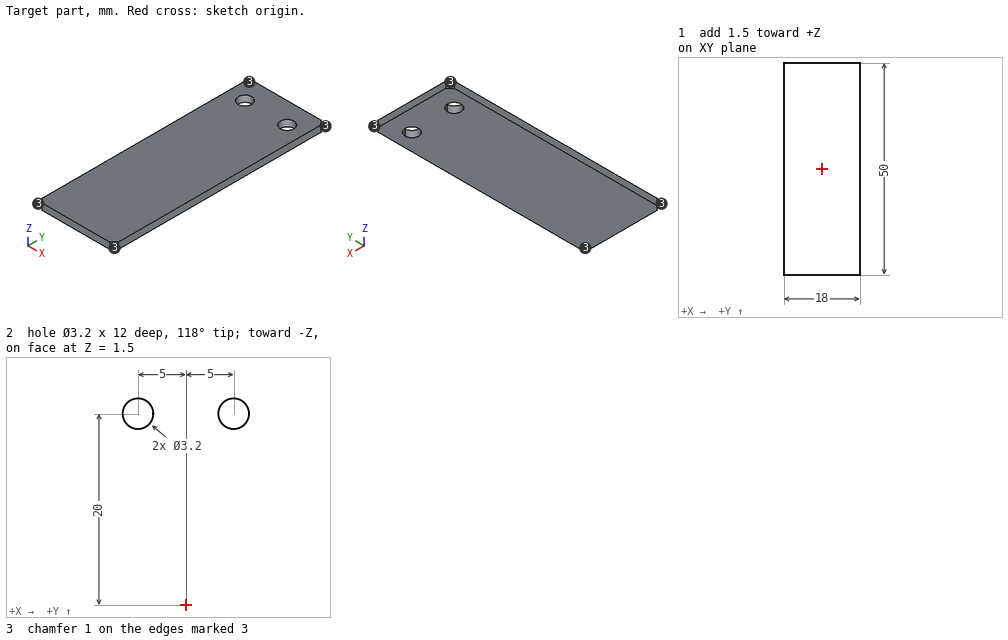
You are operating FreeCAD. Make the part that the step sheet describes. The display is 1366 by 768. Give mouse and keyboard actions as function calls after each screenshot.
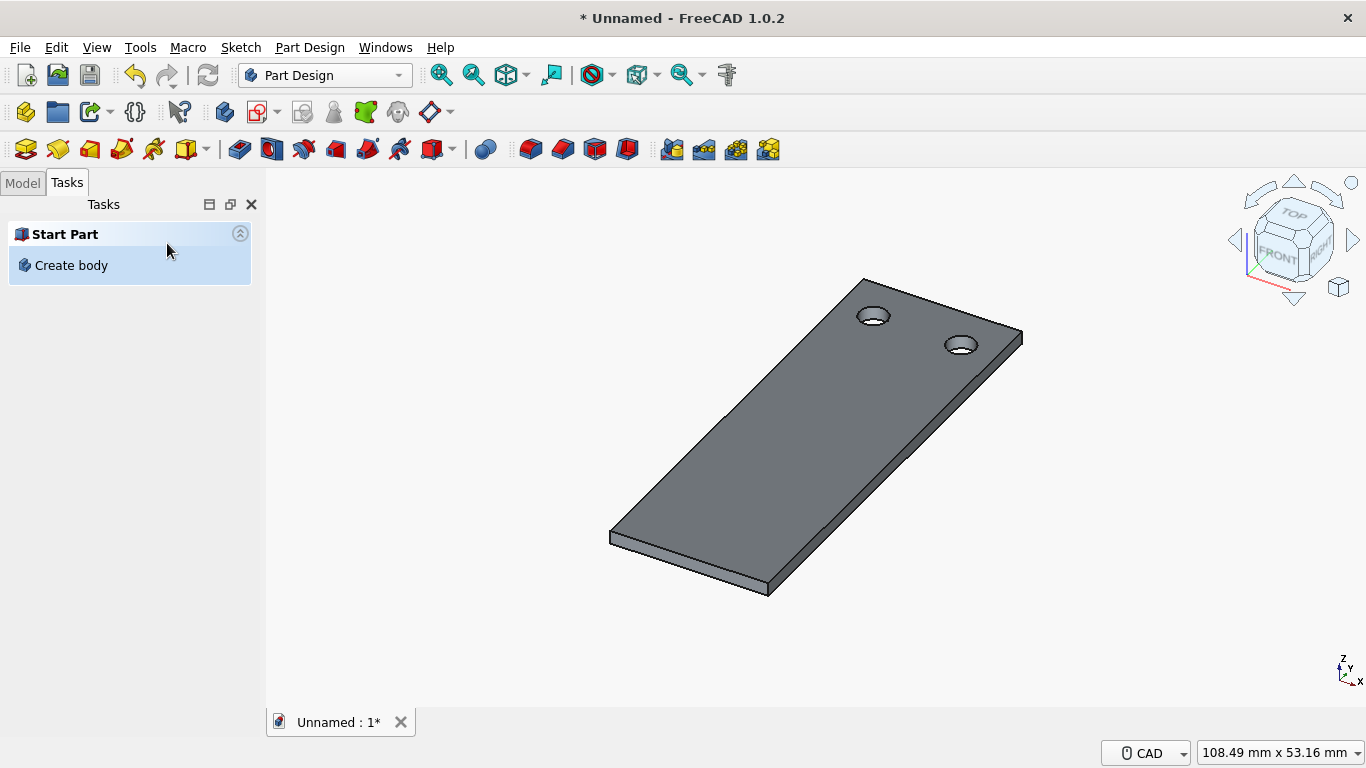
click(768, 589)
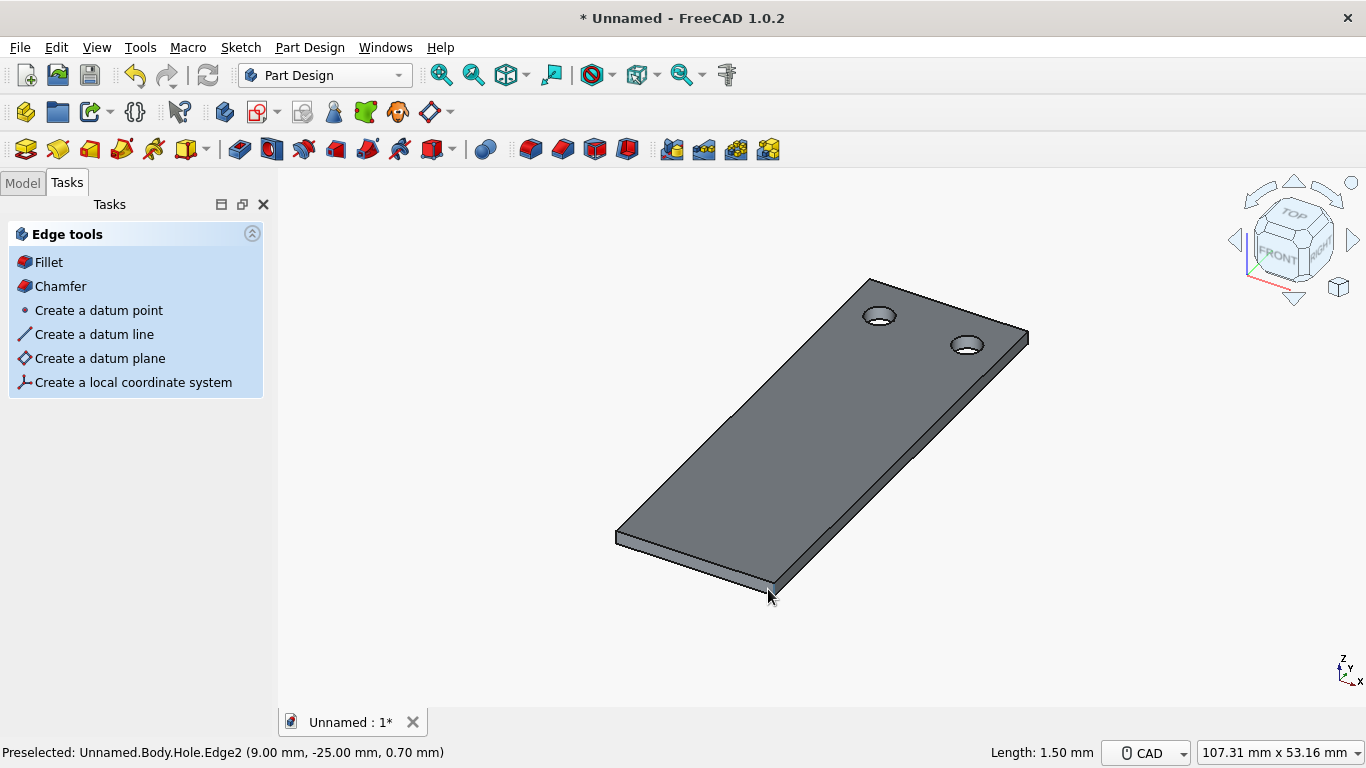
scroll(616, 536, up, 5)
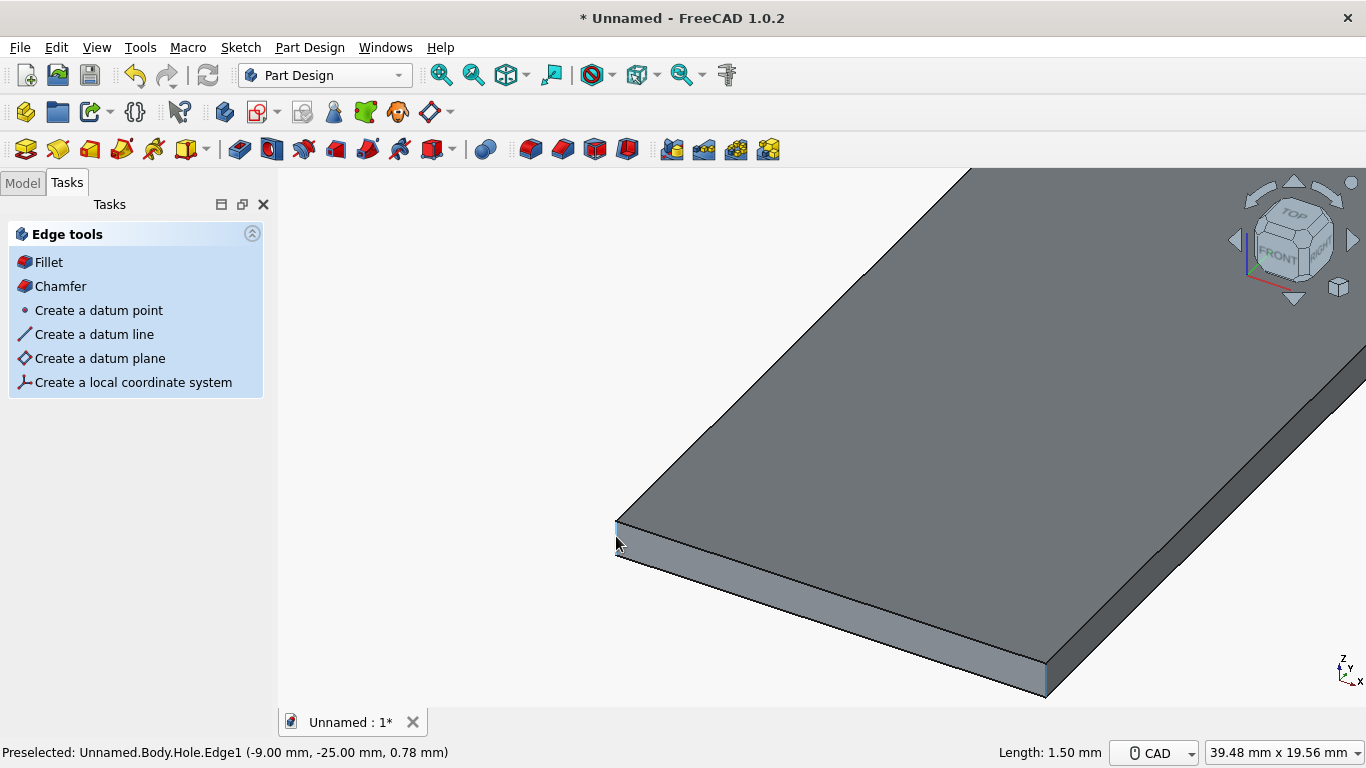
click(442, 76)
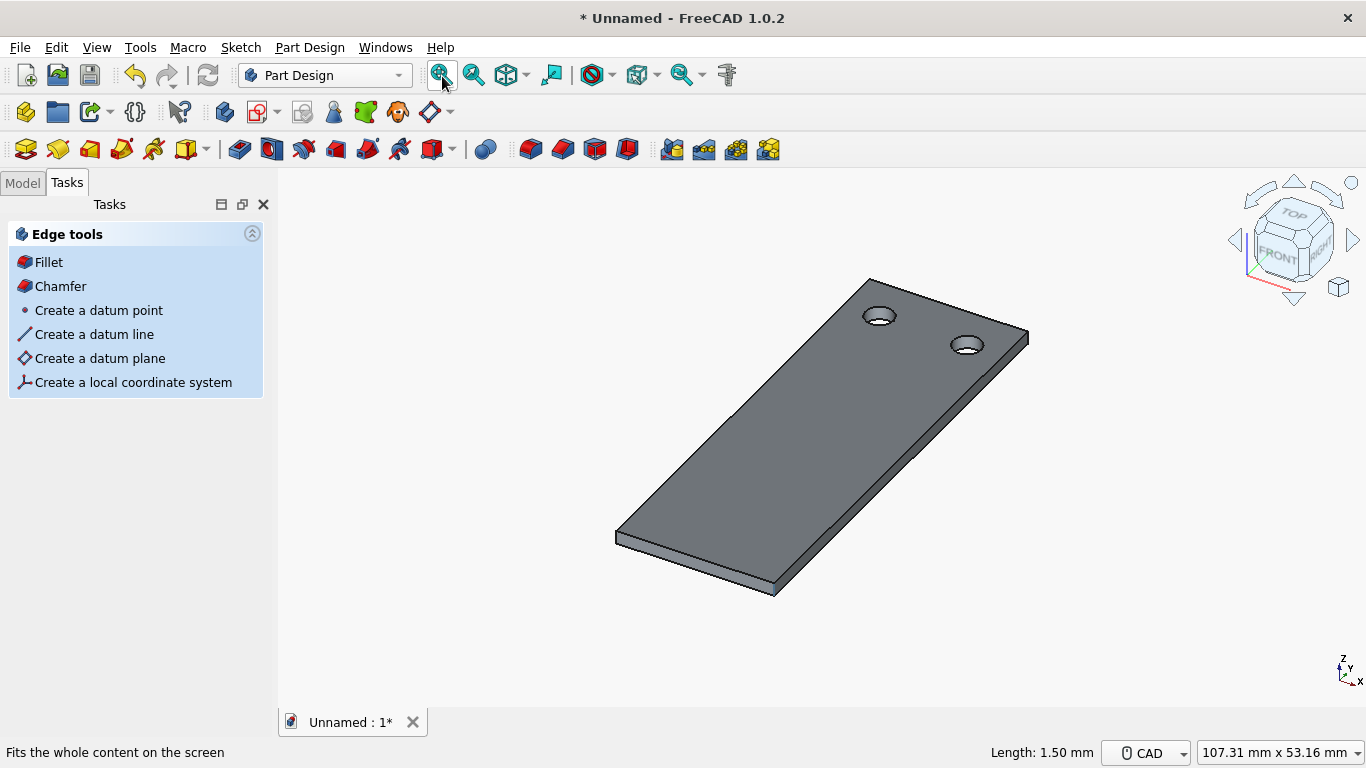
key(0)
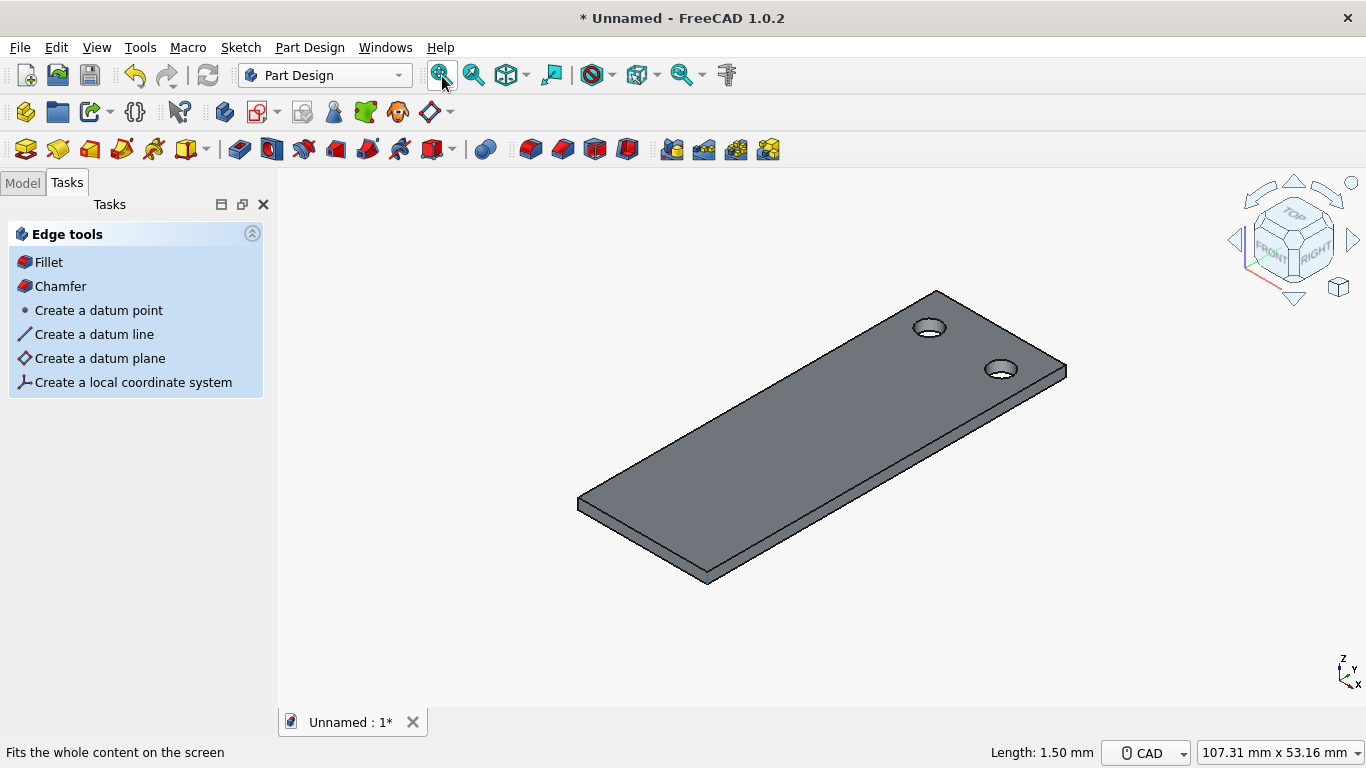
scroll(578, 503, up, 5)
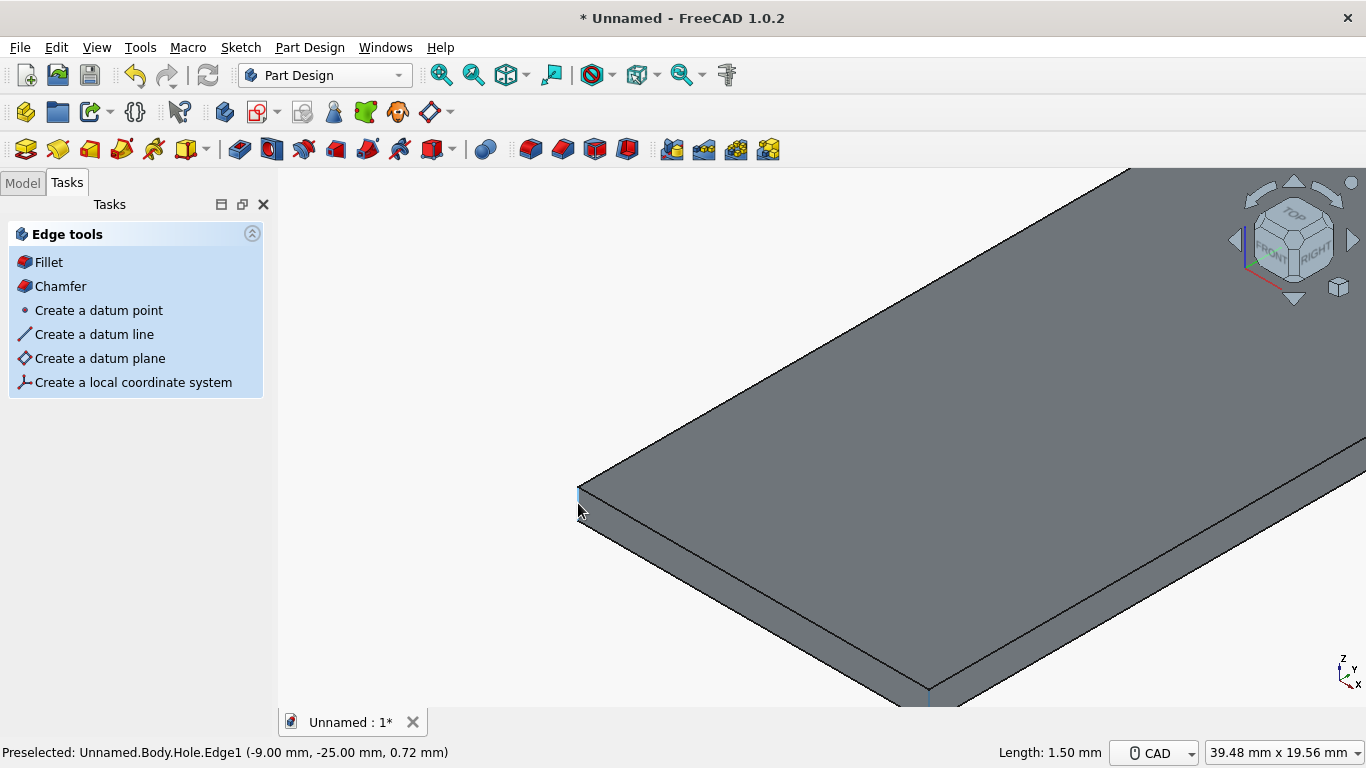
click(442, 76)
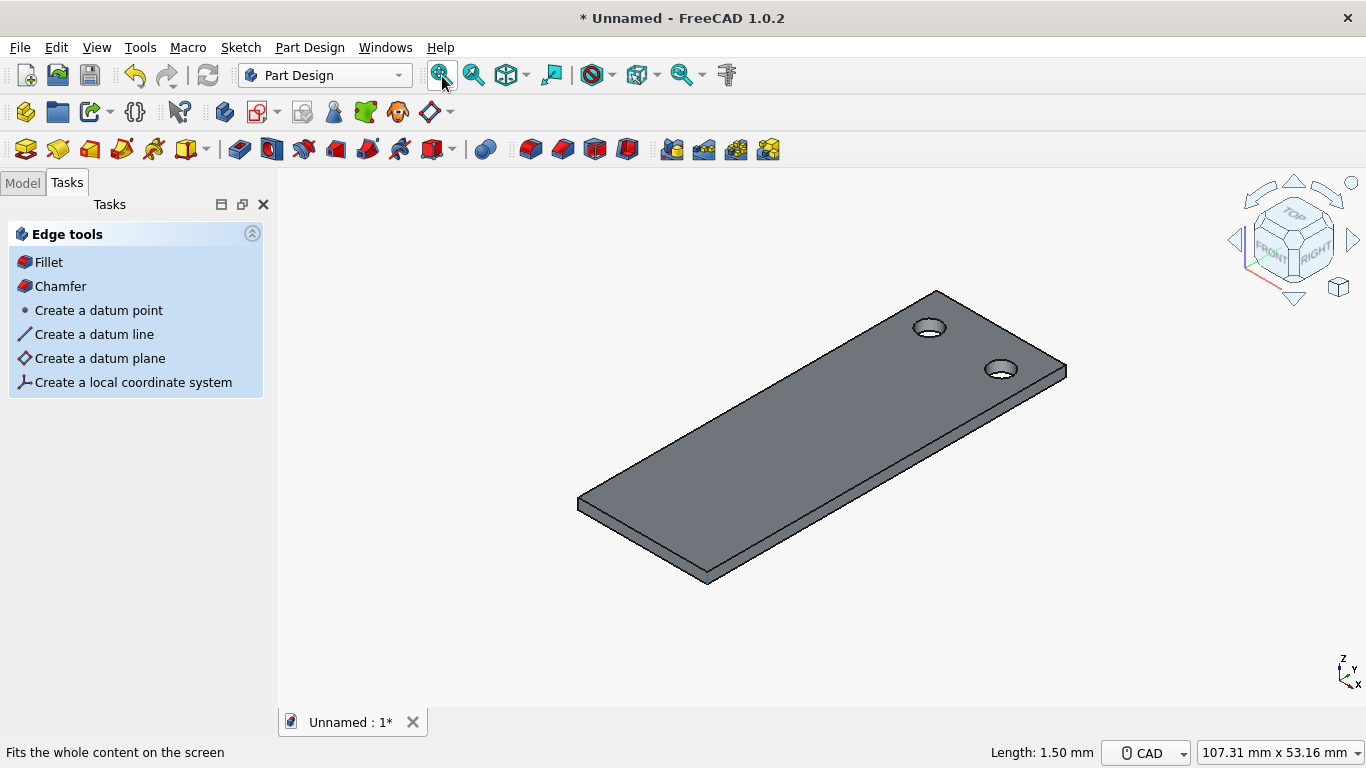
key(2)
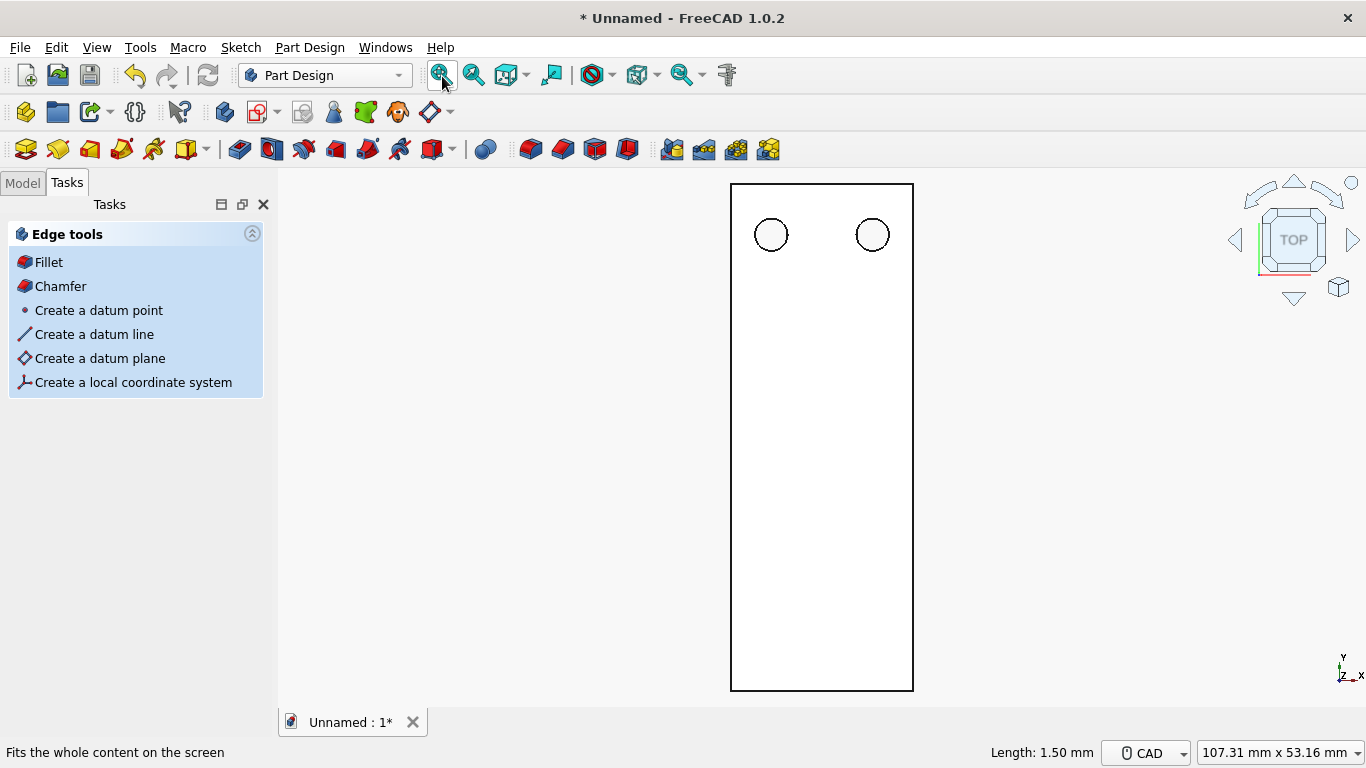
key(1)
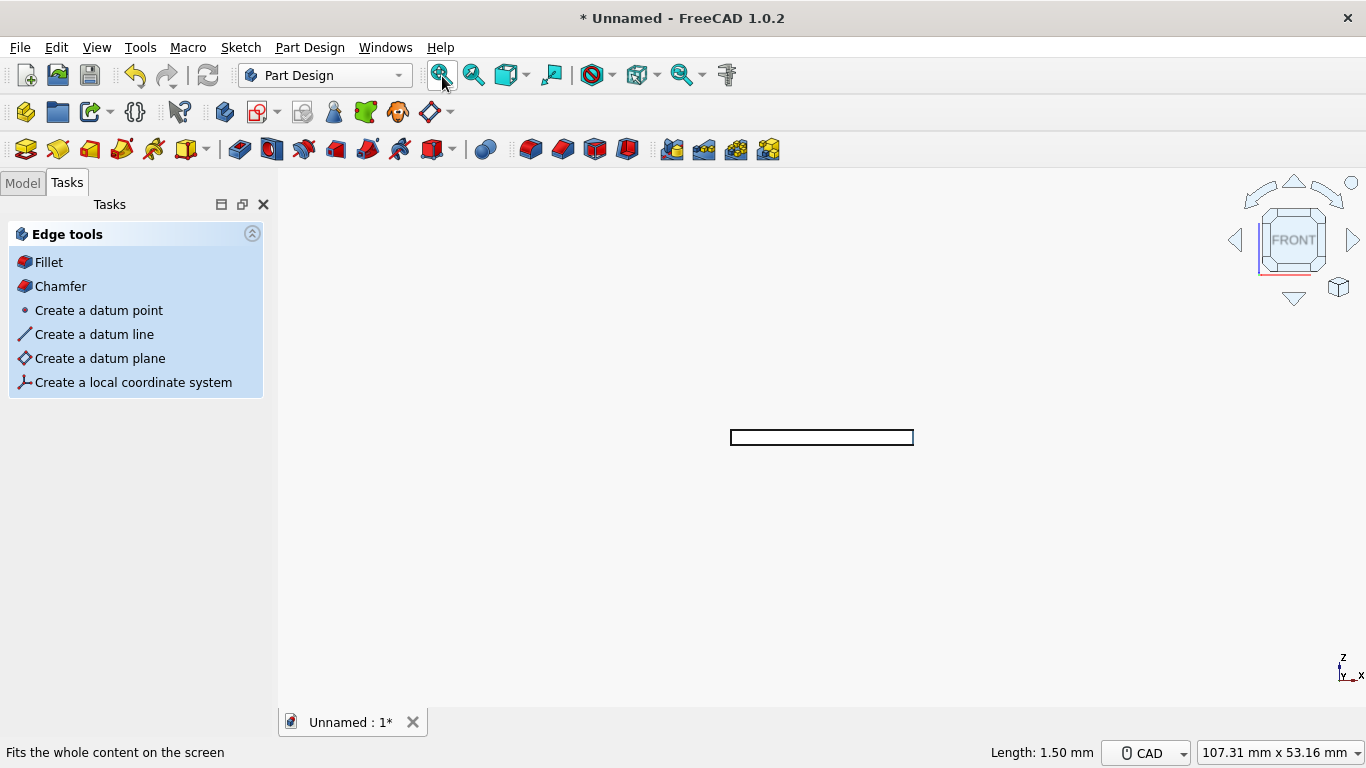
click(442, 76)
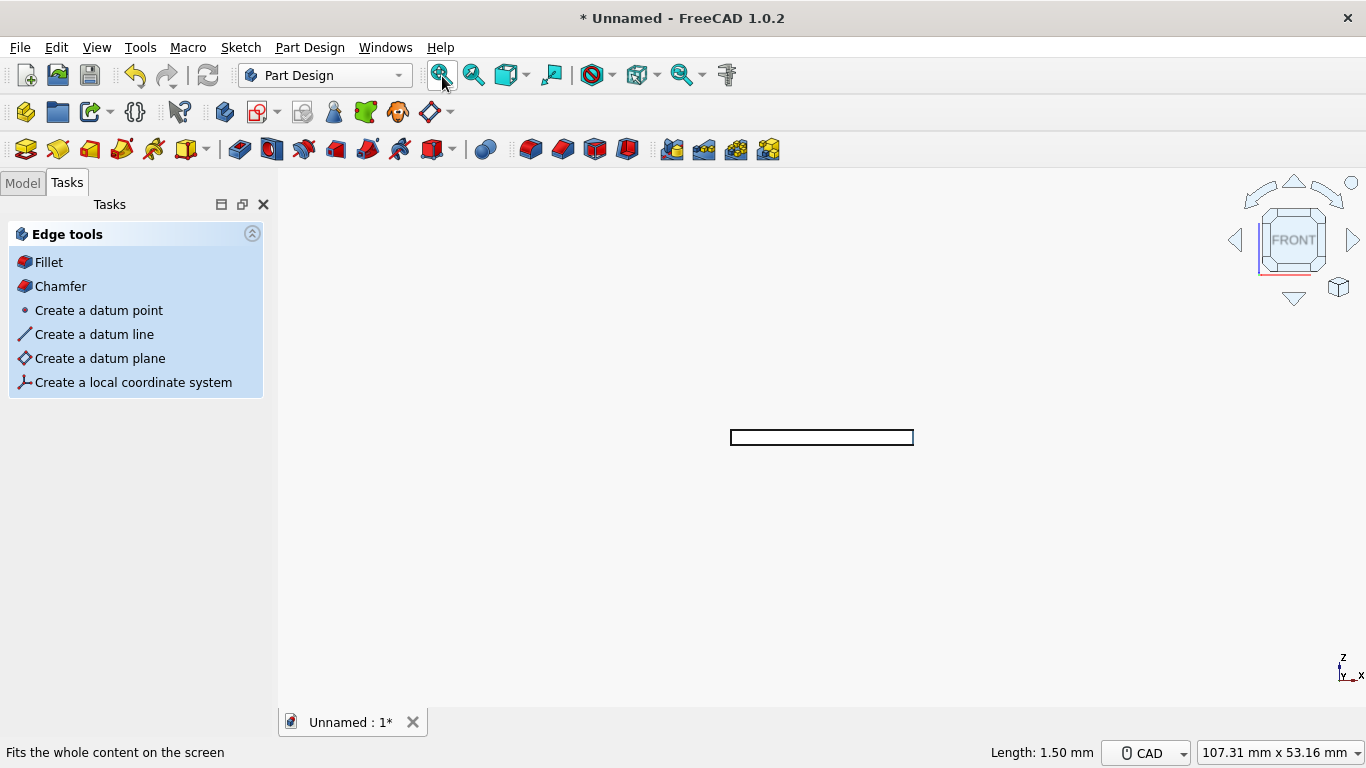
click(731, 437, ctrl)